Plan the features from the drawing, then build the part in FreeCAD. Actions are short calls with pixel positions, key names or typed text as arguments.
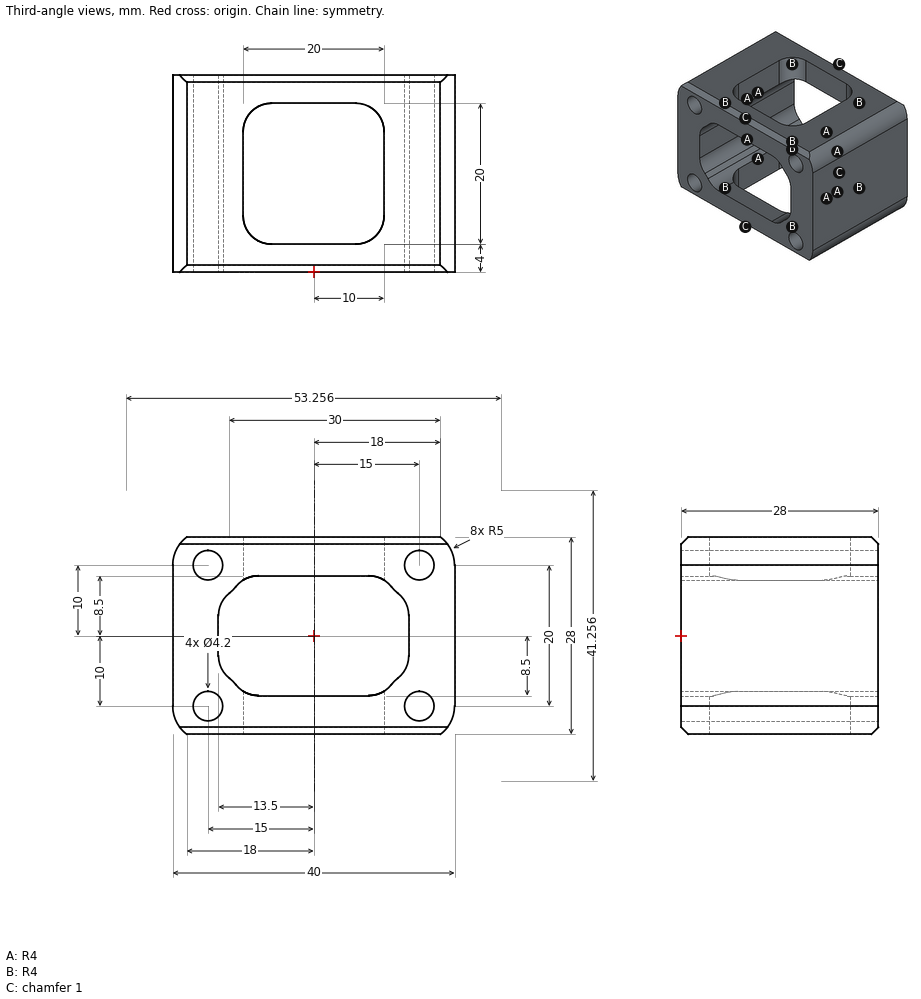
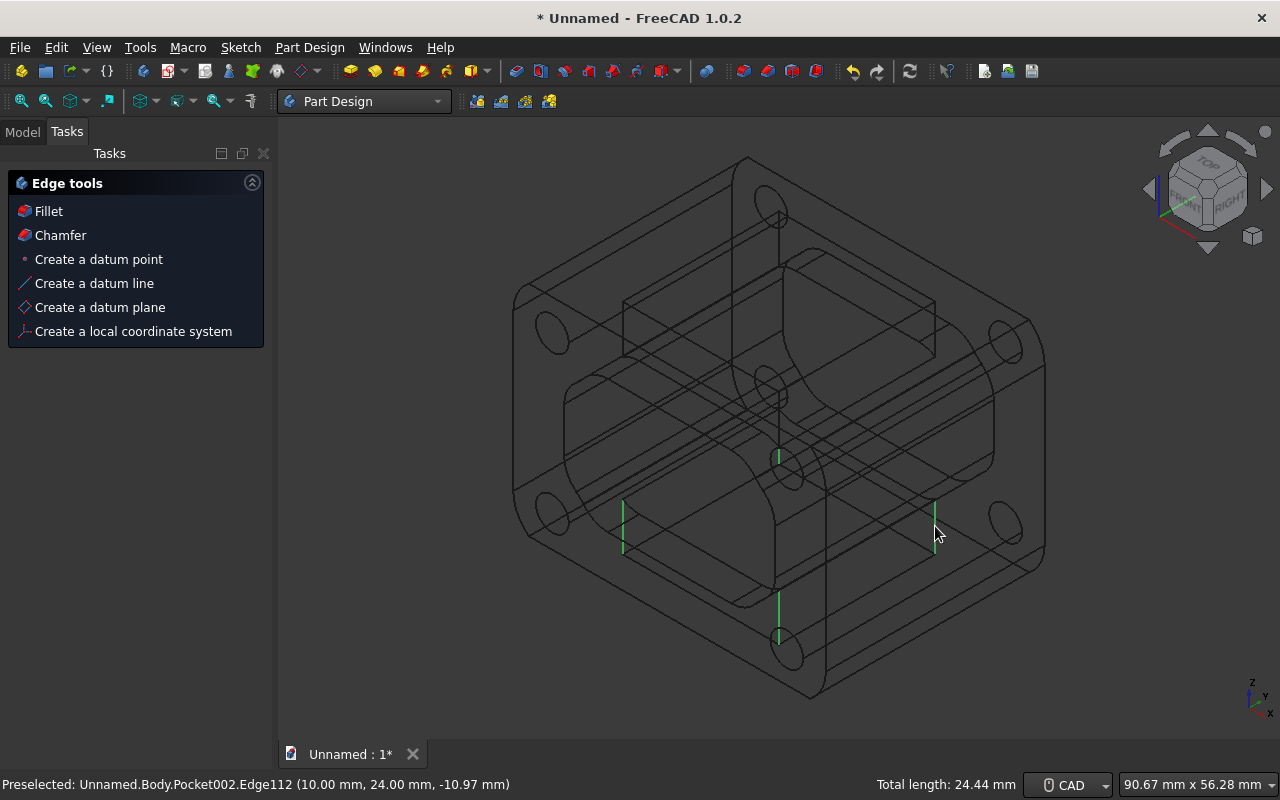
click(779, 418, ctrl)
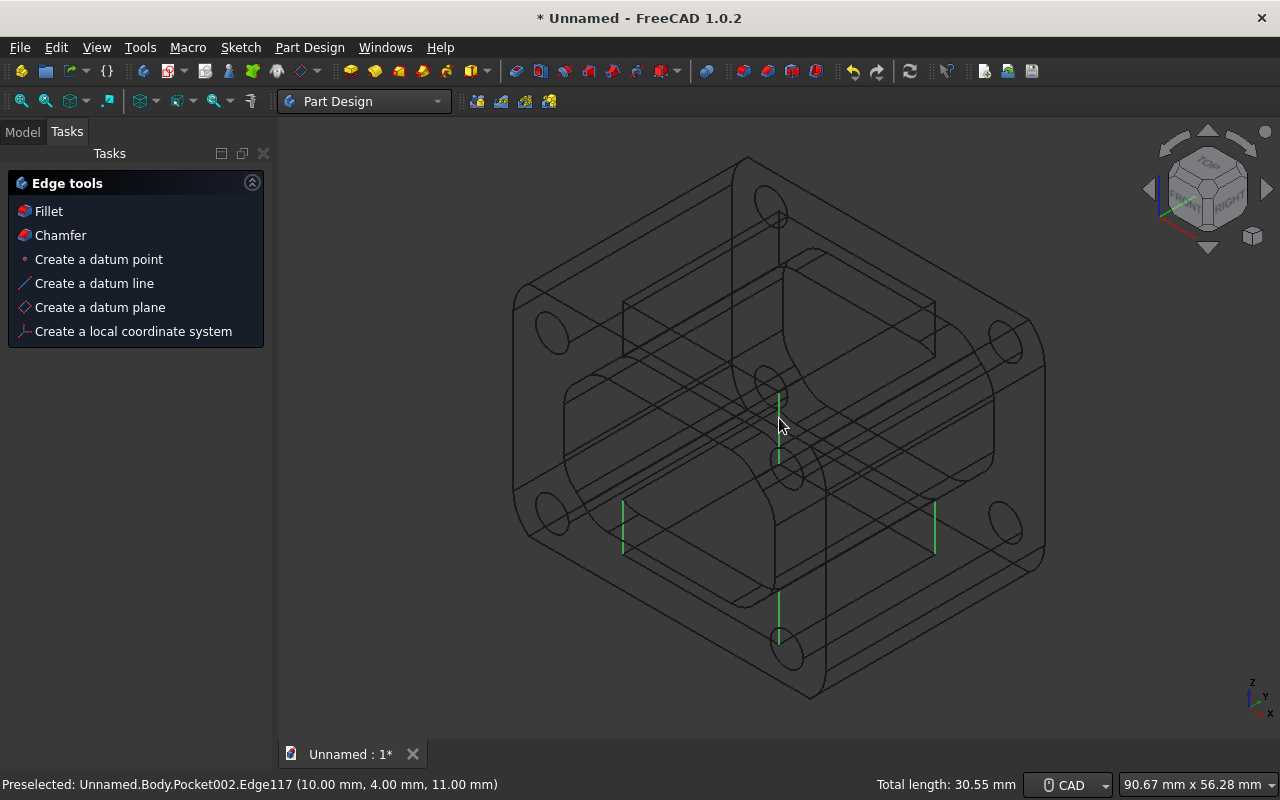
click(623, 328, ctrl)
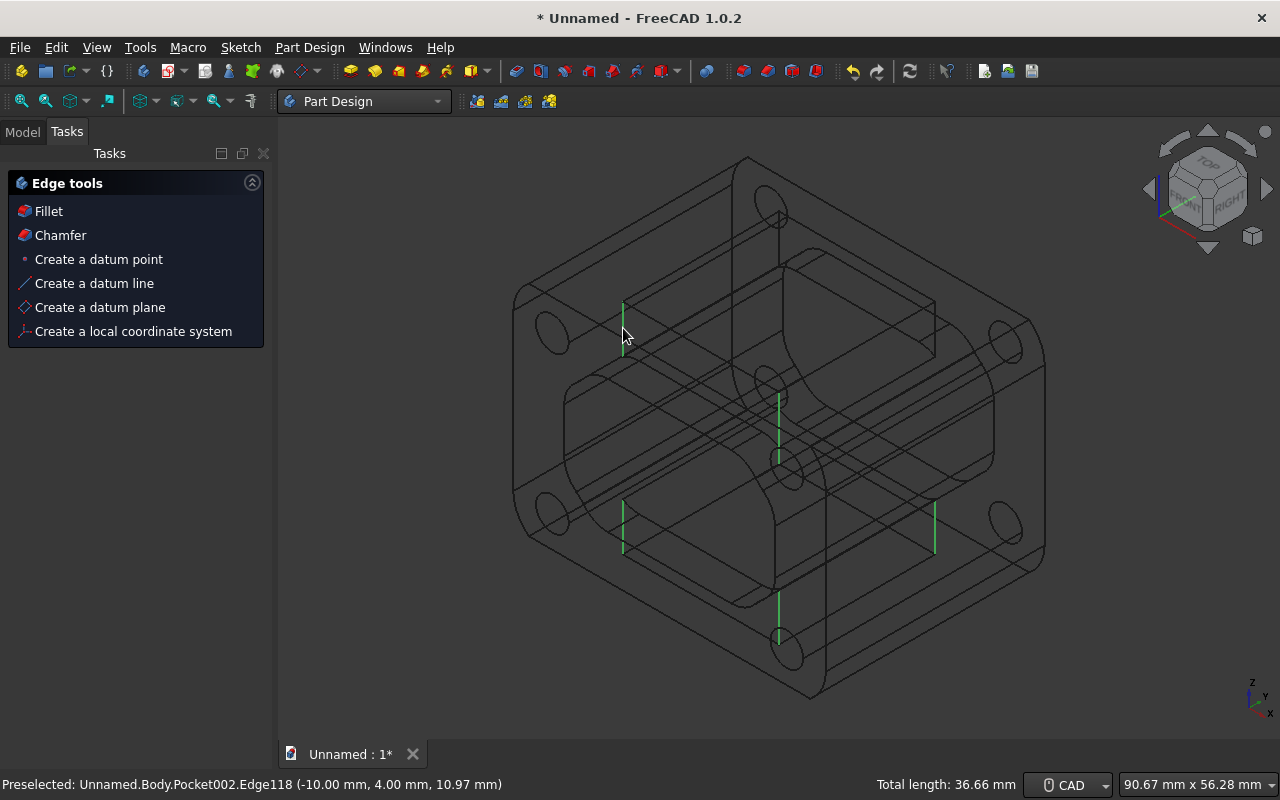
click(779, 238, ctrl)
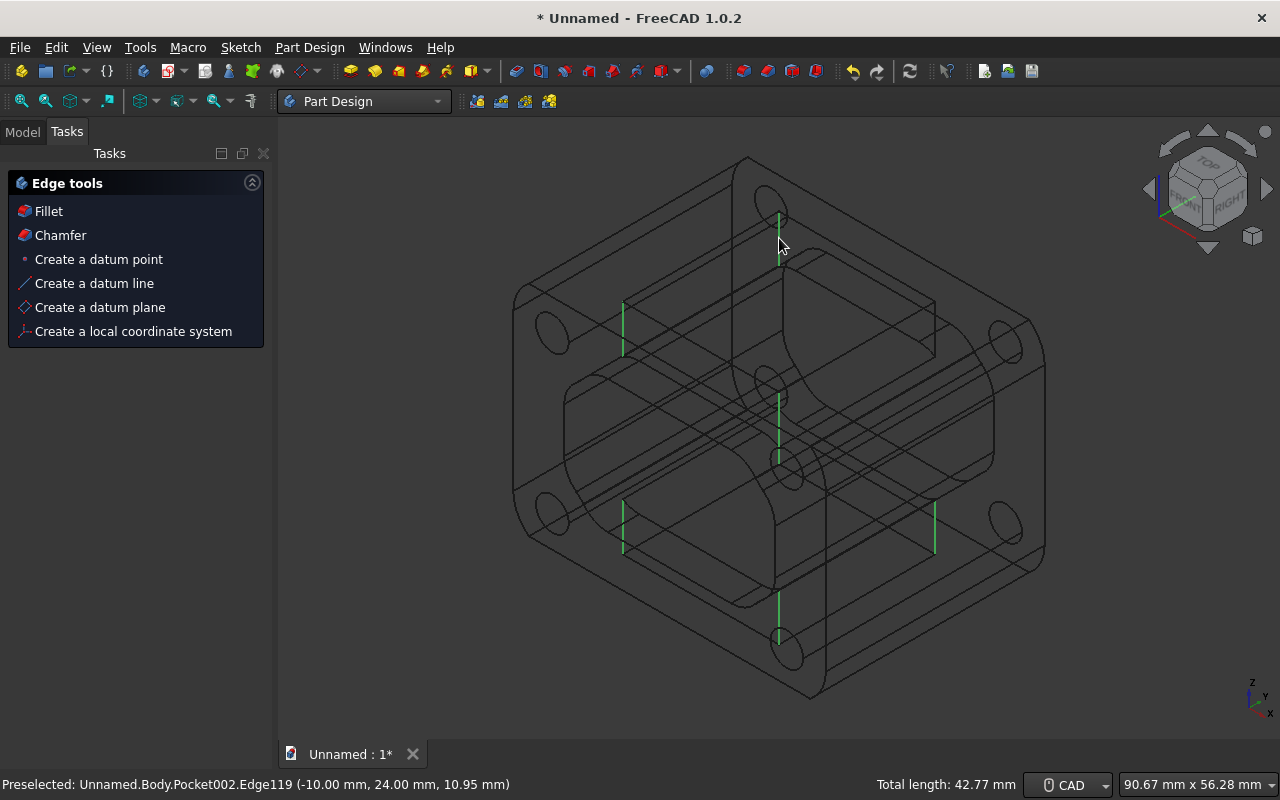
click(935, 328, ctrl)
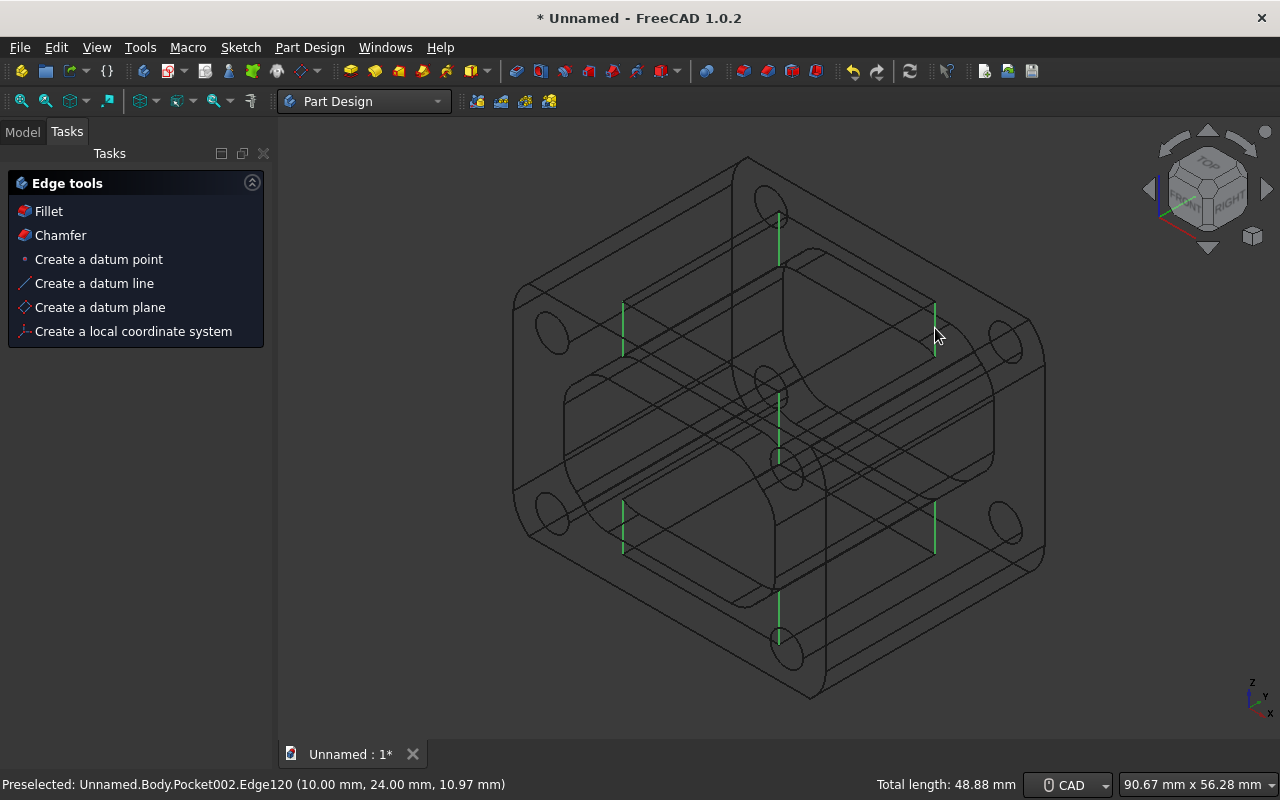
key(v)
key(1)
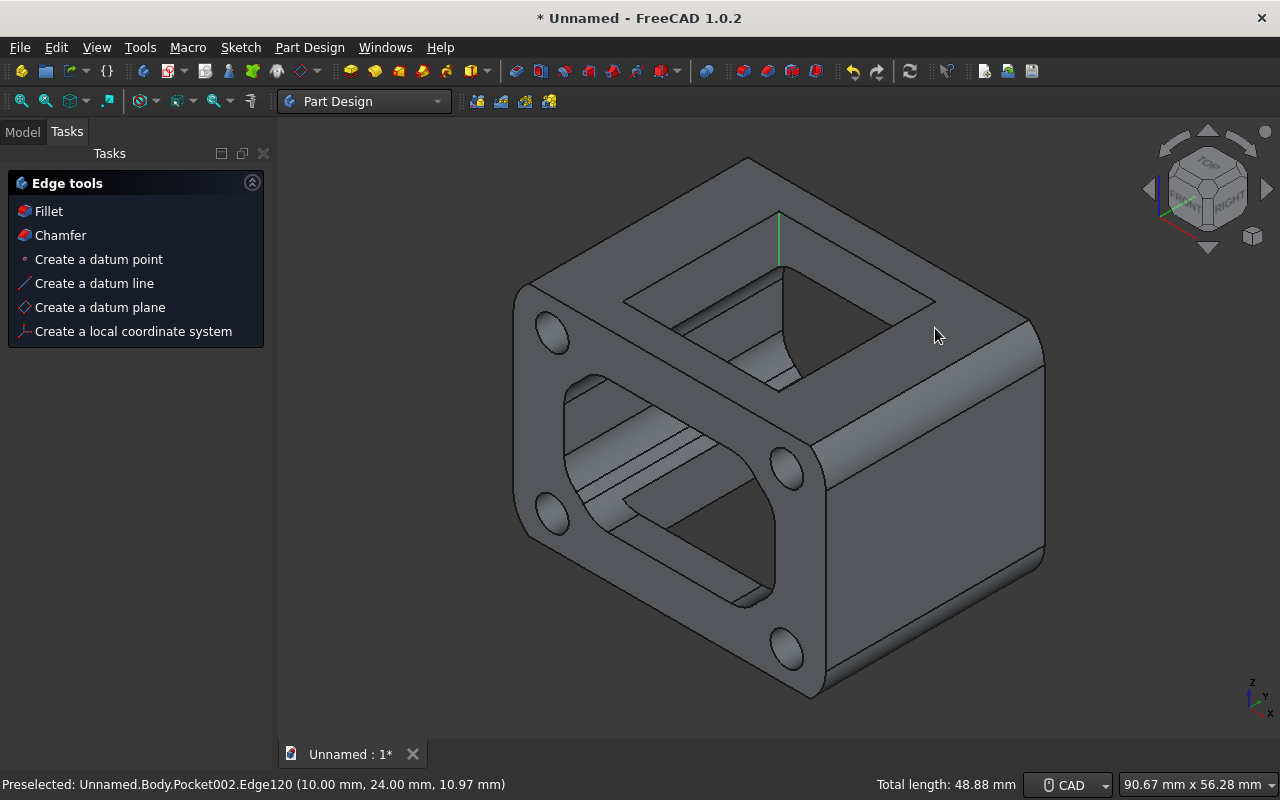
click(744, 72)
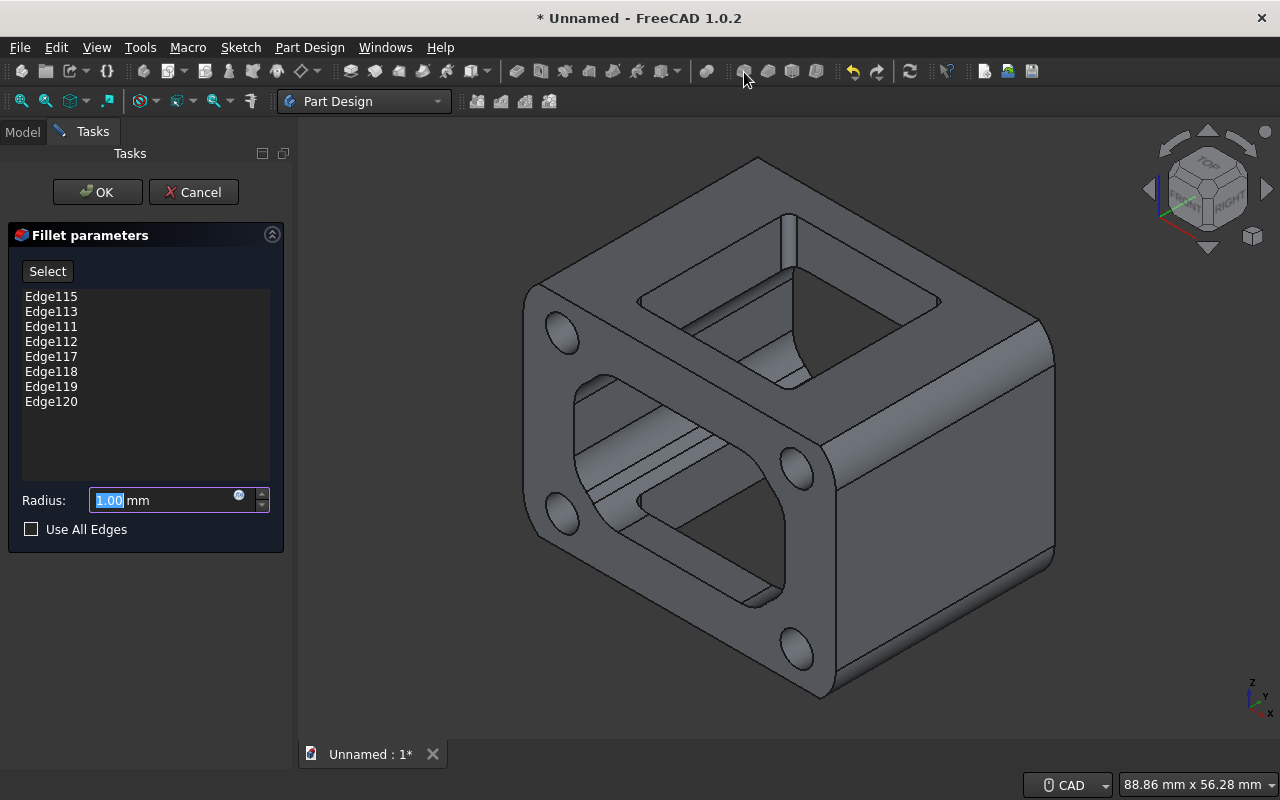
text(4)
key(Tab)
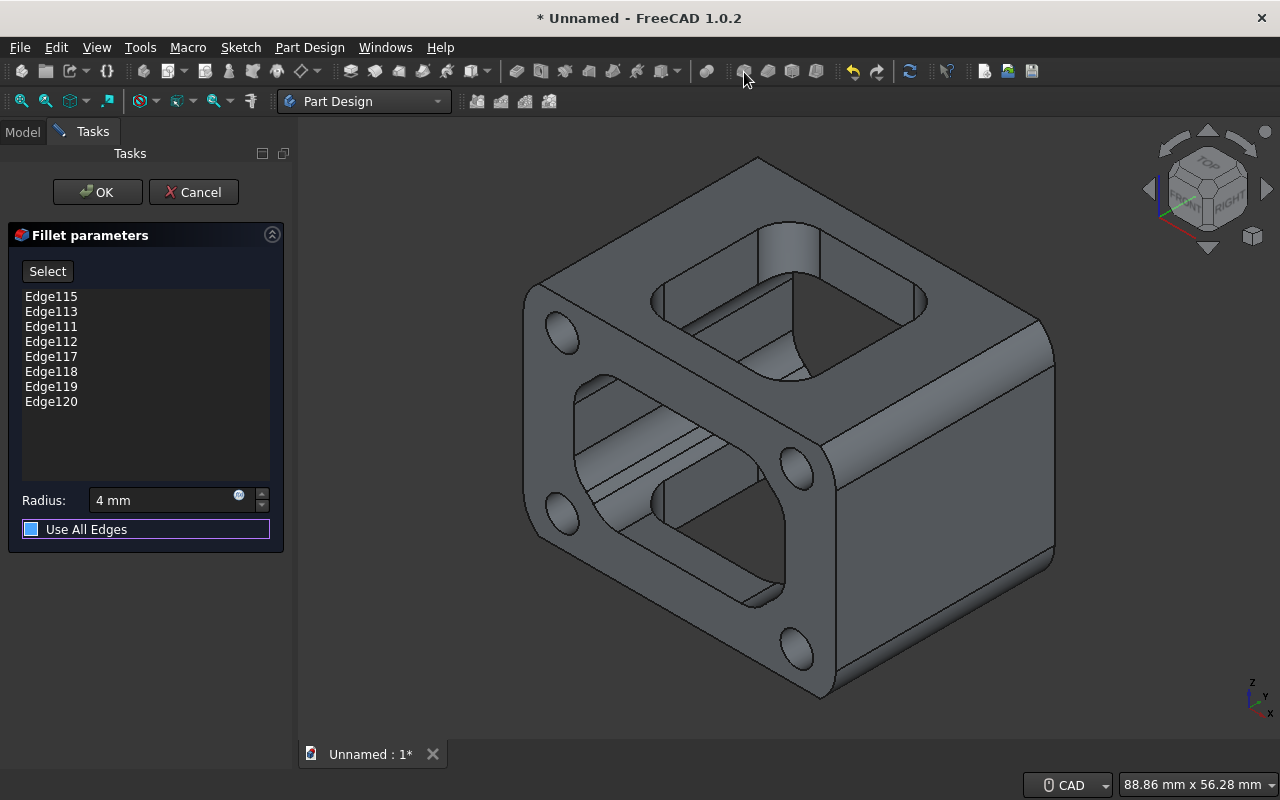
click(98, 192)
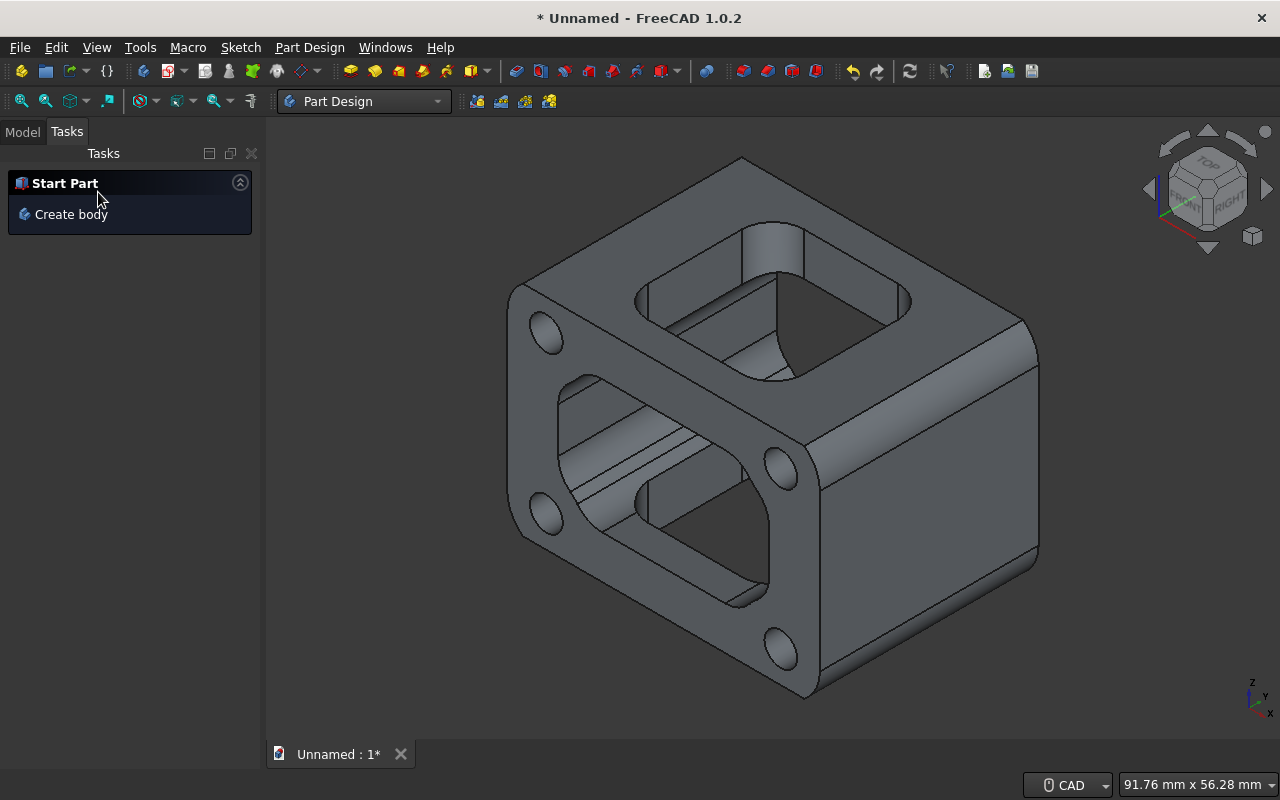
click(664, 364)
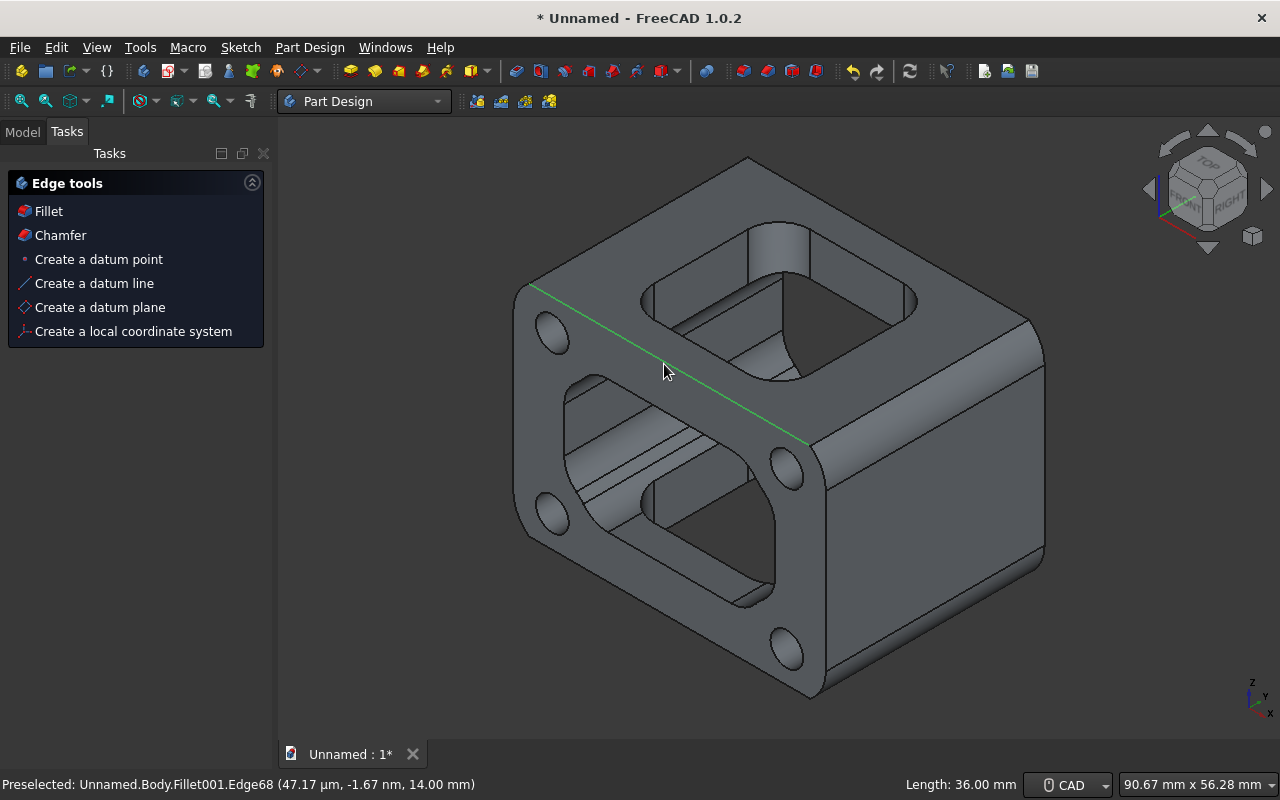
key(2)